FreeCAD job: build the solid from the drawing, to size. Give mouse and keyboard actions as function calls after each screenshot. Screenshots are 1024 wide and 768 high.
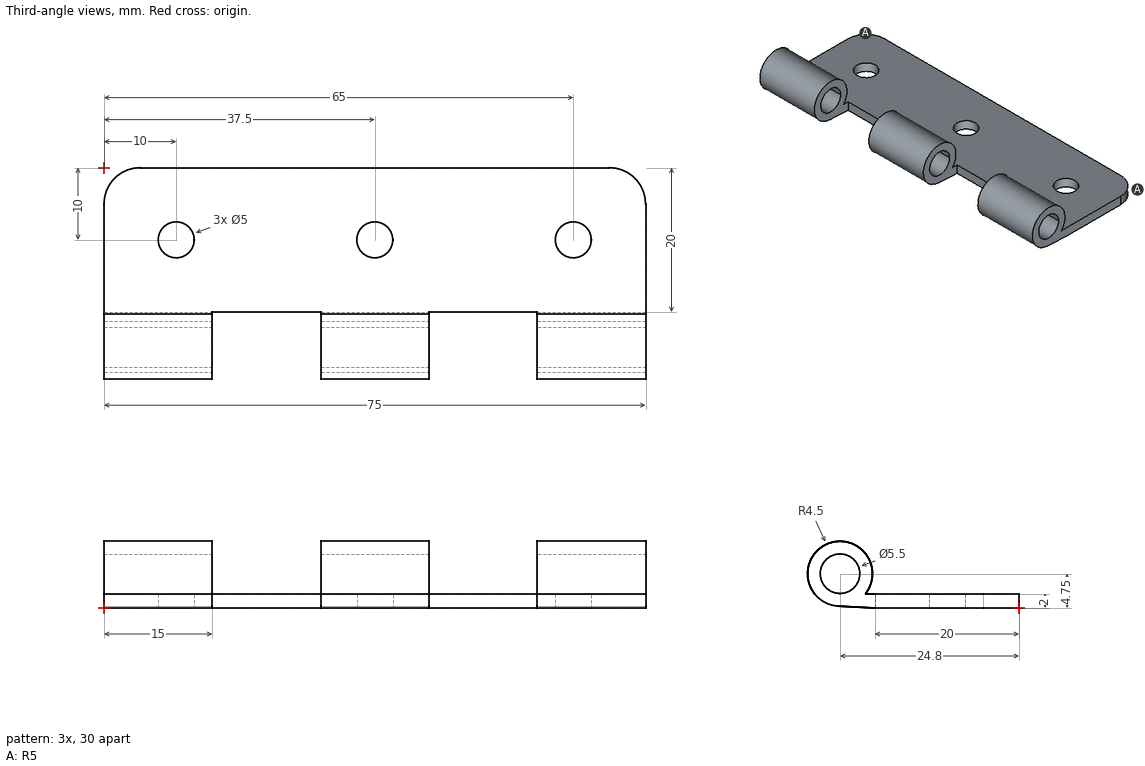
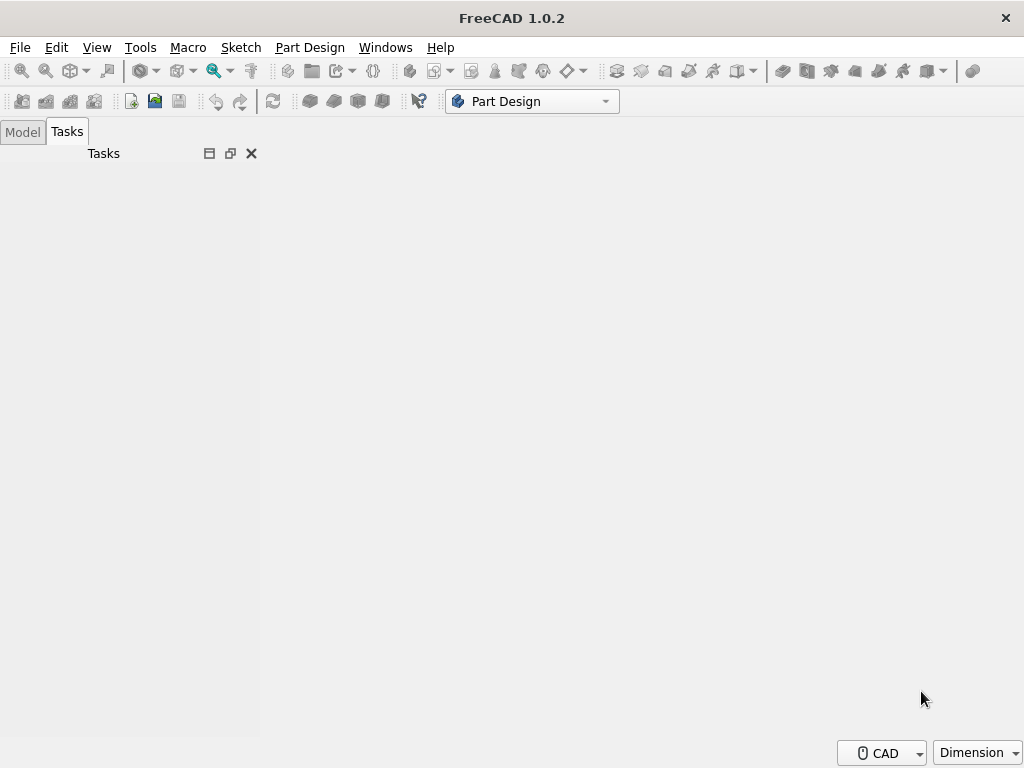
click(132, 102)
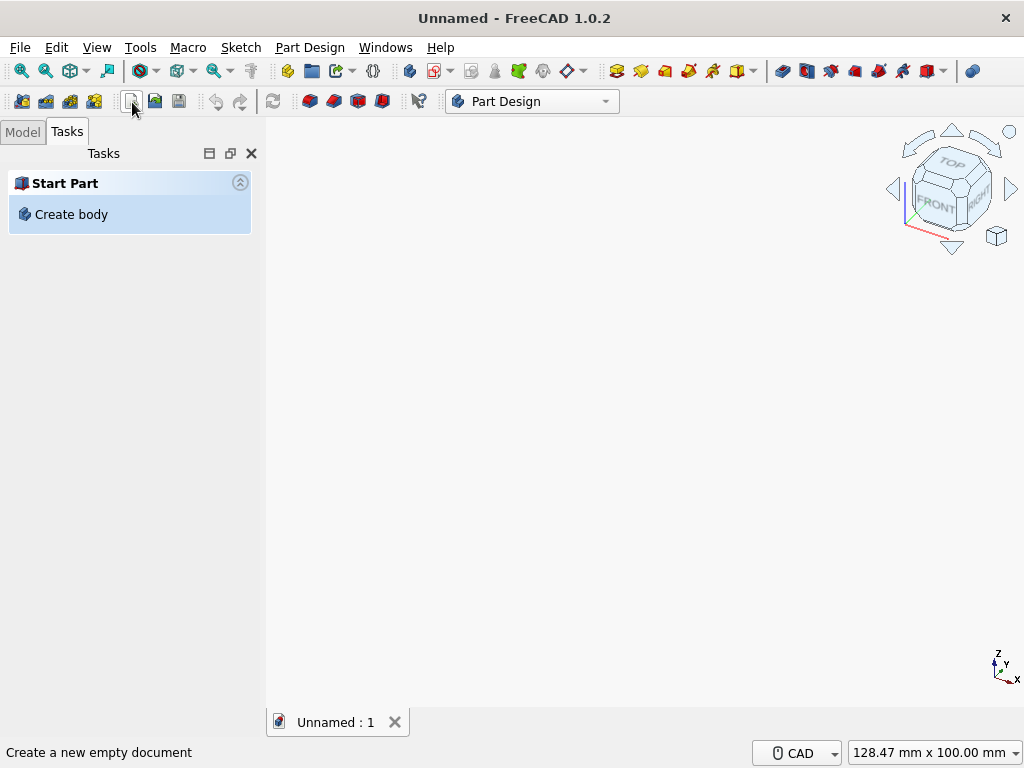
click(434, 72)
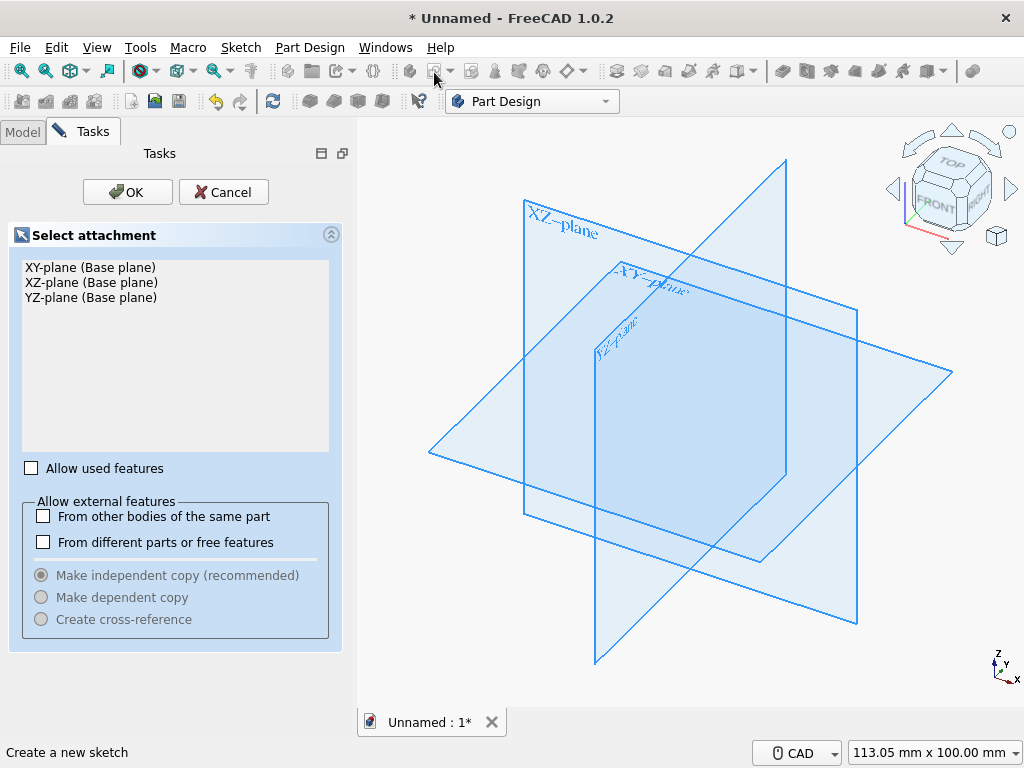
click(82, 268)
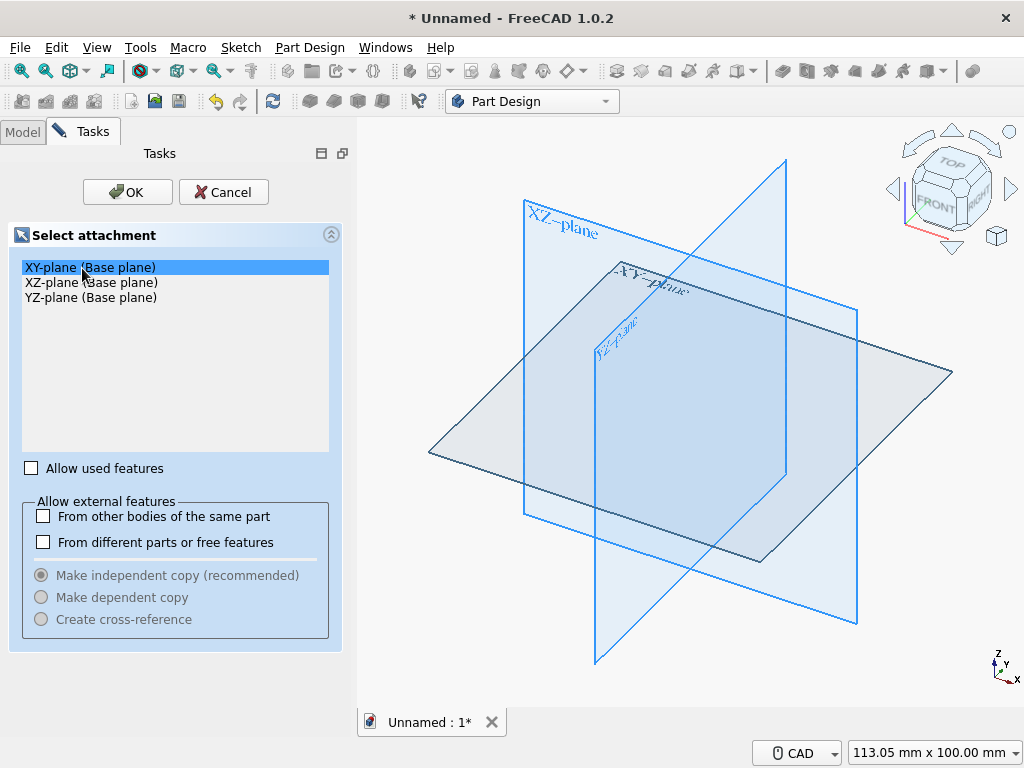
click(128, 192)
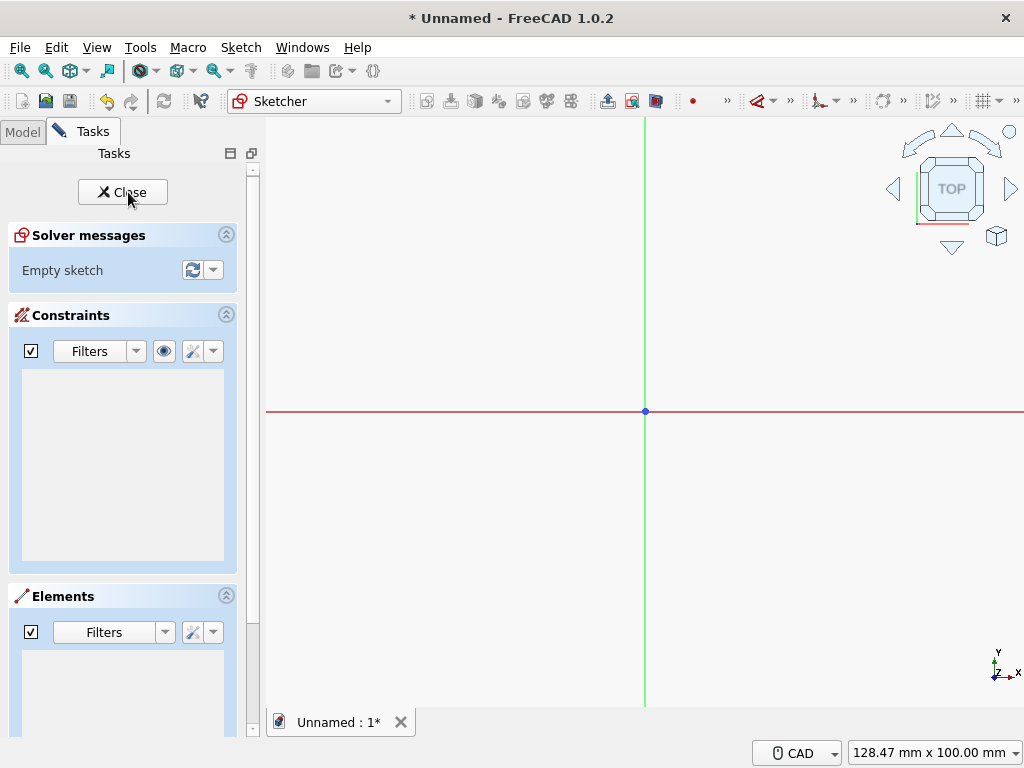
scroll(294, 292, down, 2)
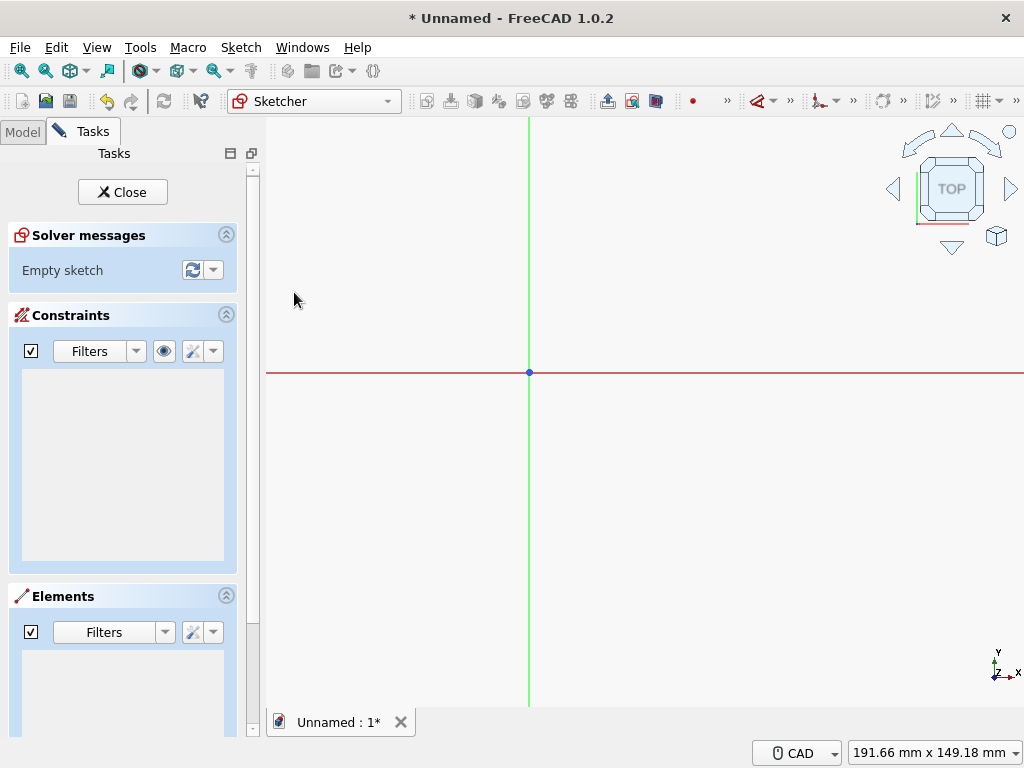
key(g)
key(r)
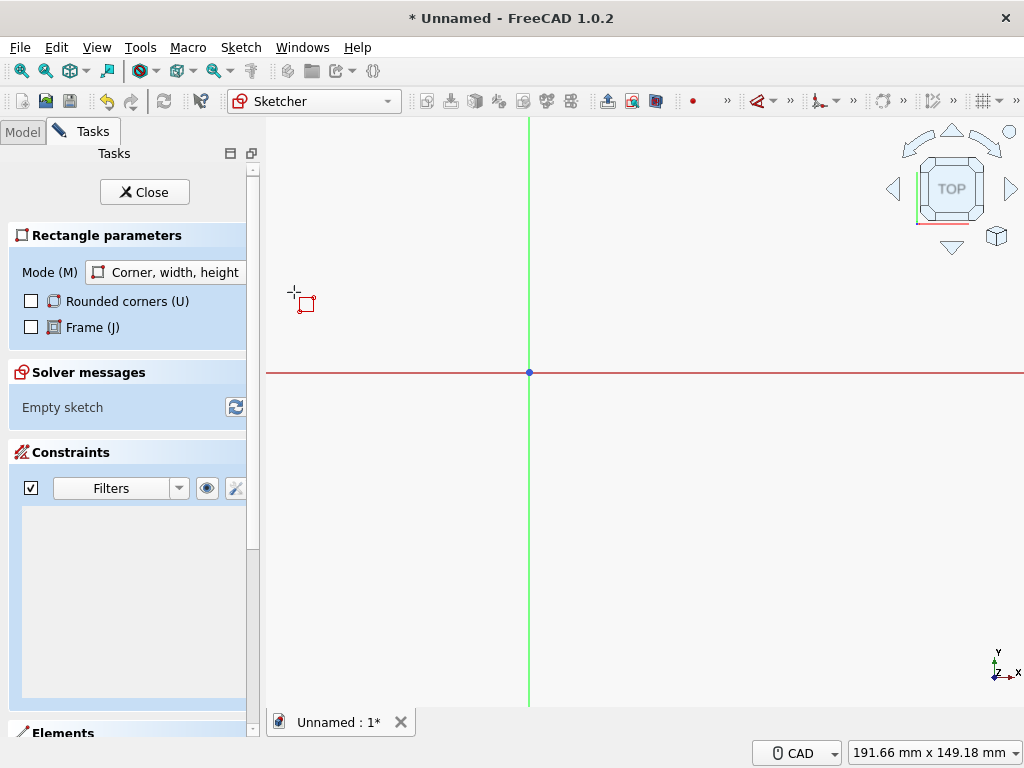
click(529, 373)
move(826, 452)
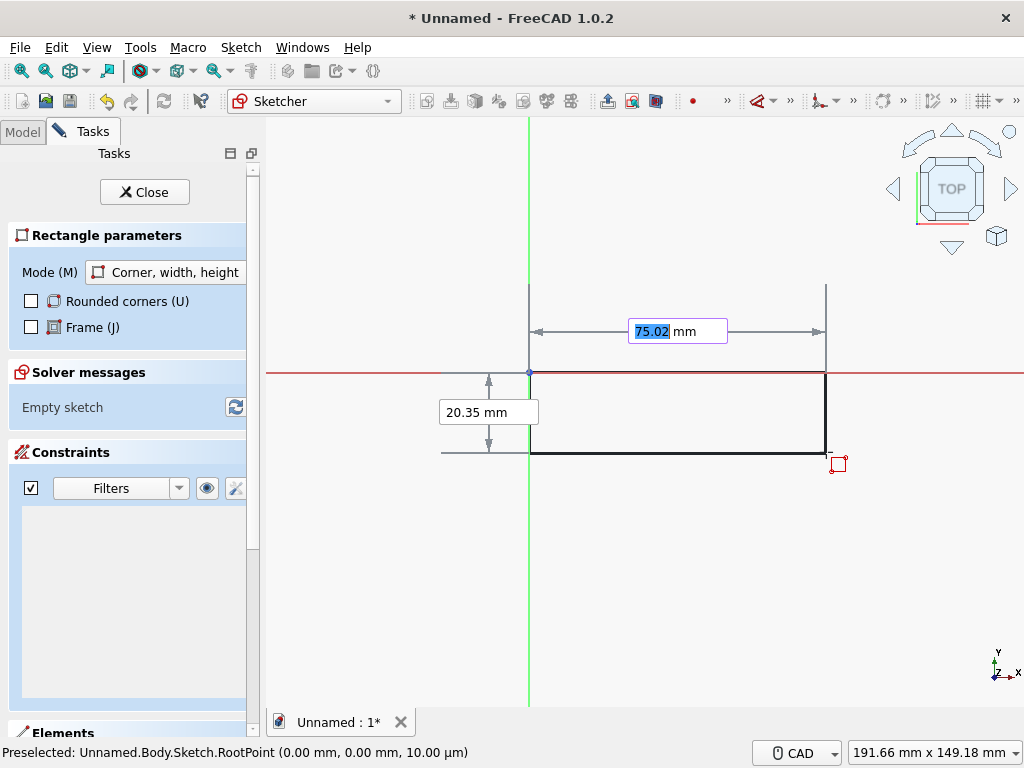
text(75)
key(Tab)
text(20)
key(Return)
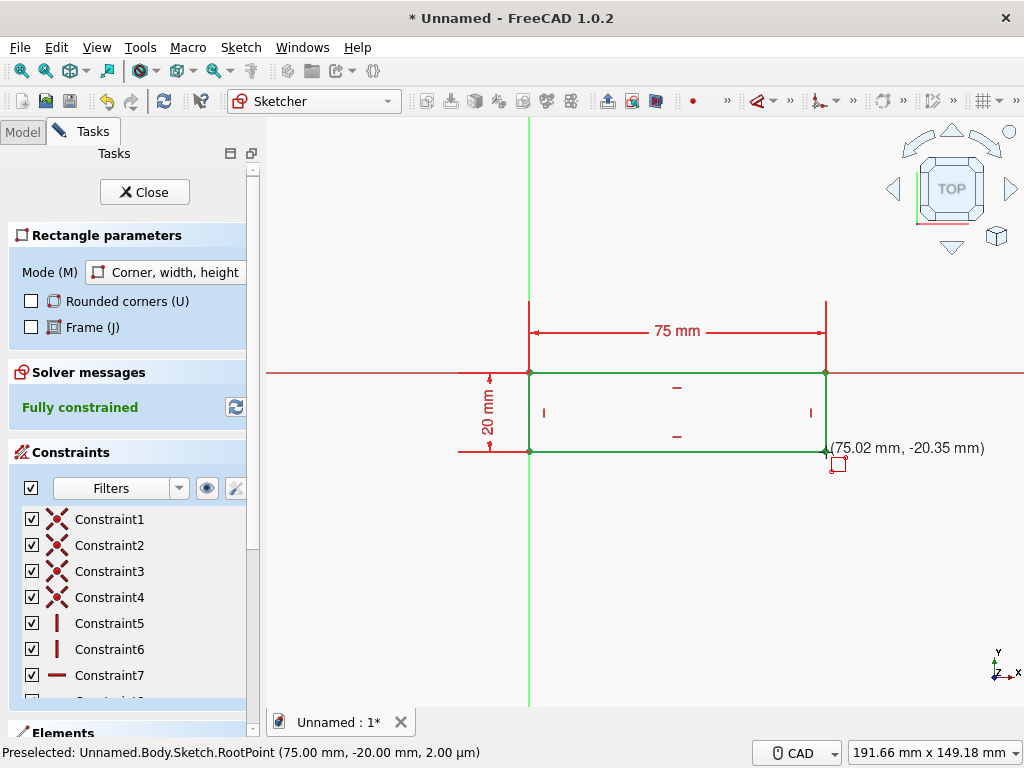
key(g)
key(c)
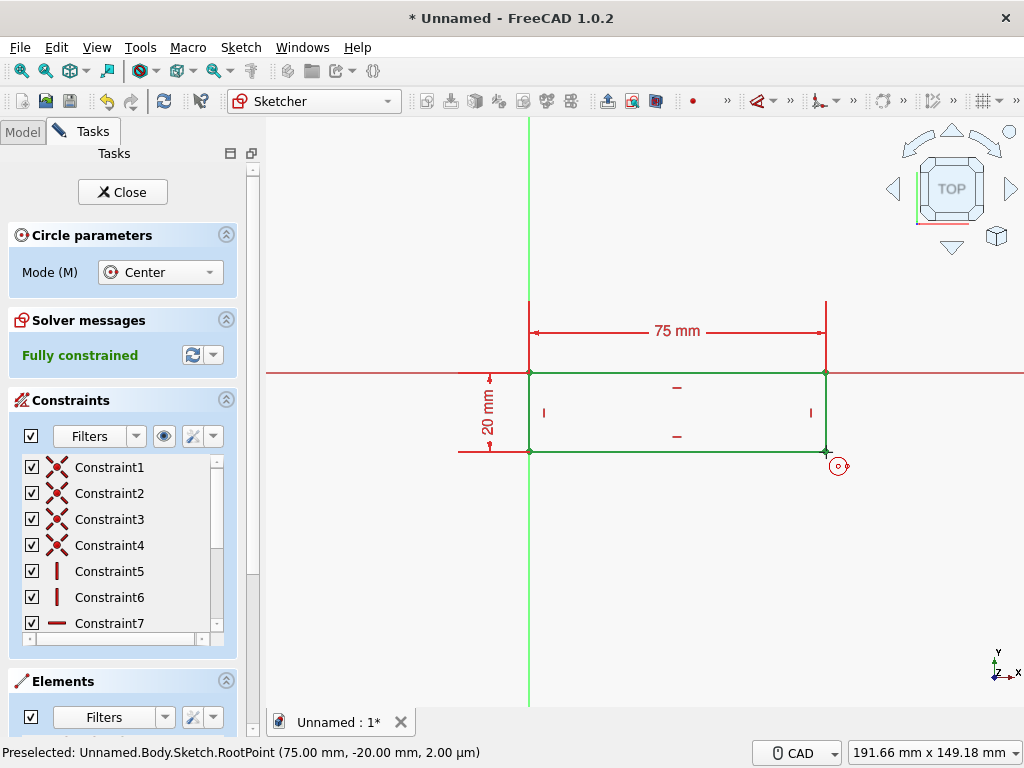
scroll(569, 412, up, 5)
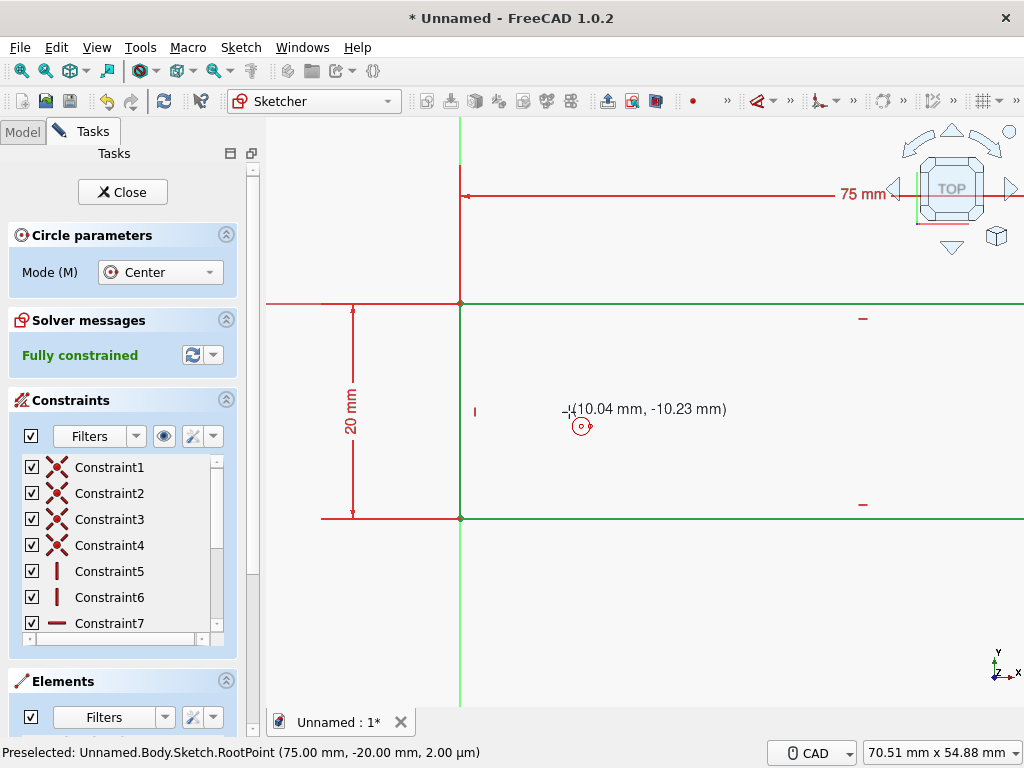
click(568, 411)
move(587, 392)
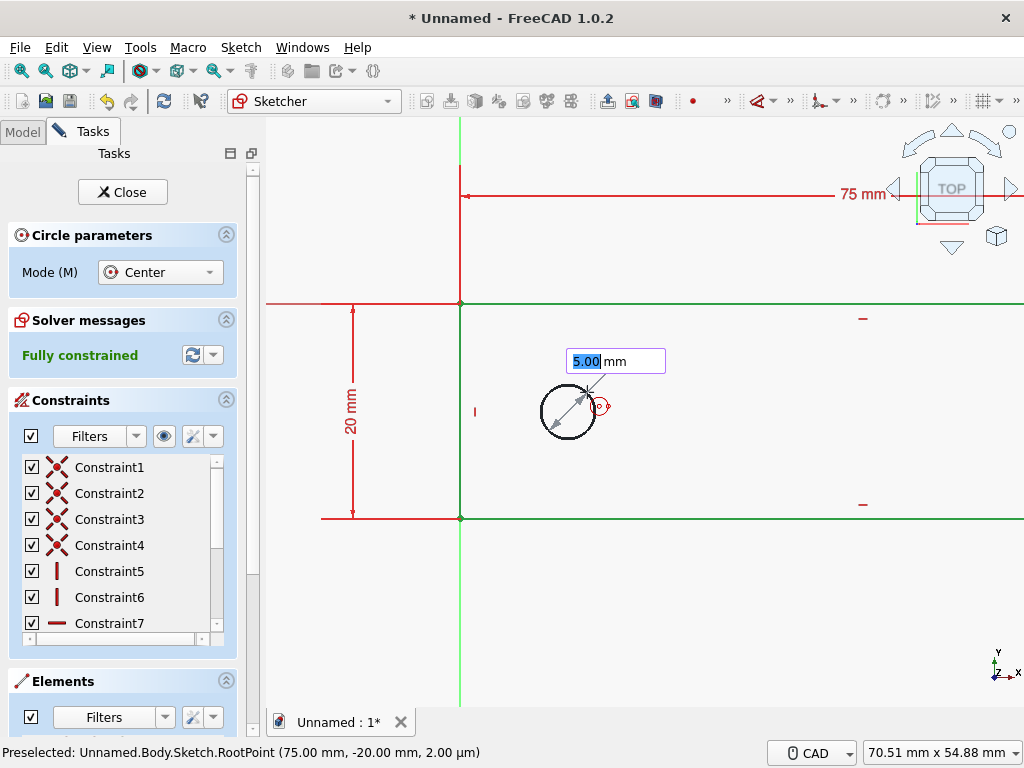
text(5)
key(Return)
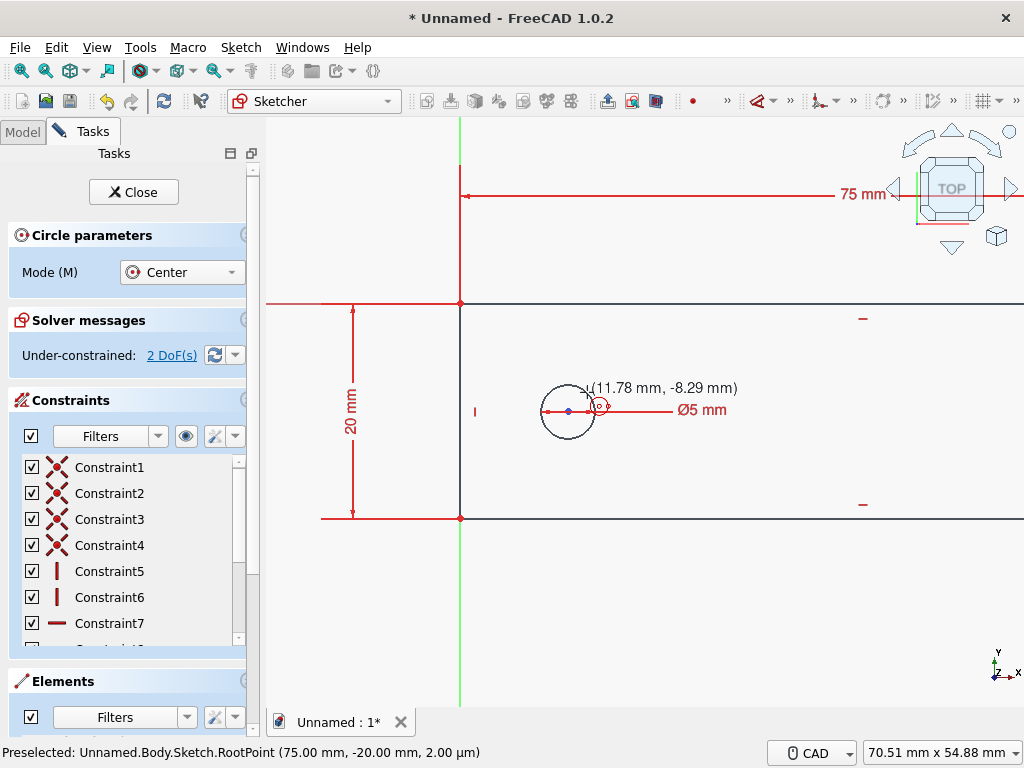
scroll(342, 413, down, 4)